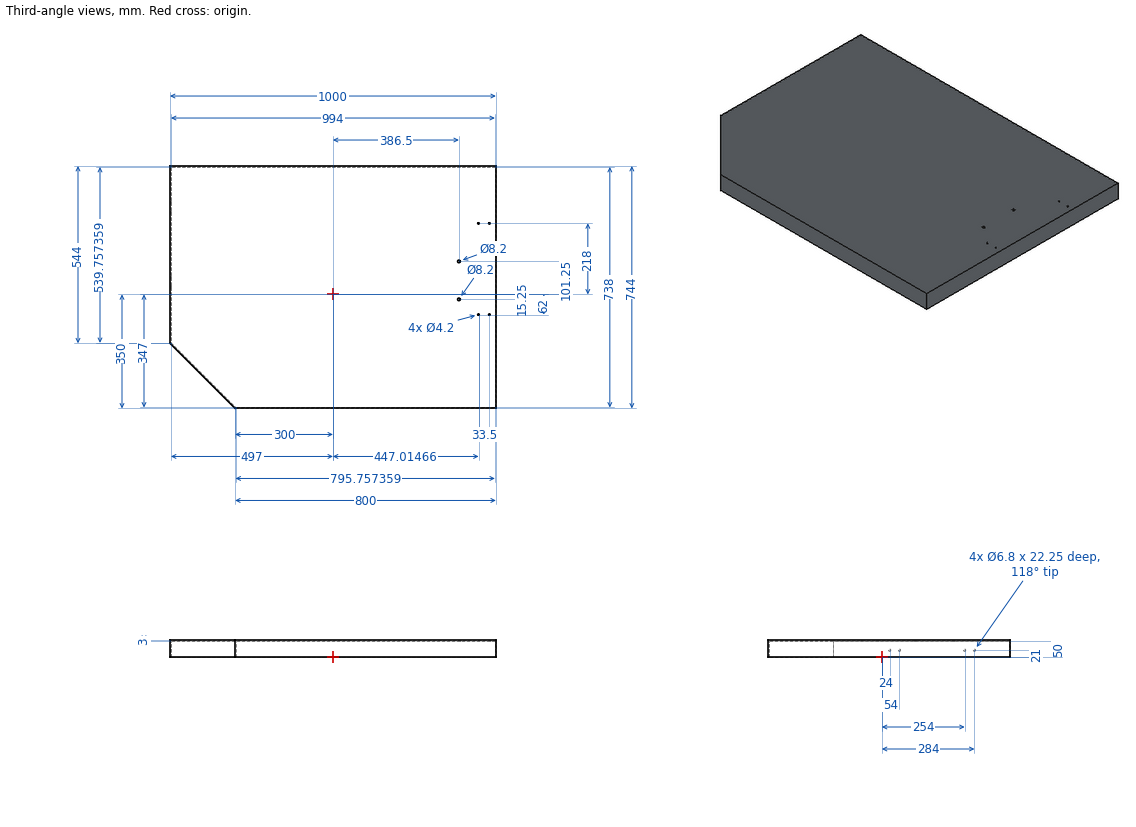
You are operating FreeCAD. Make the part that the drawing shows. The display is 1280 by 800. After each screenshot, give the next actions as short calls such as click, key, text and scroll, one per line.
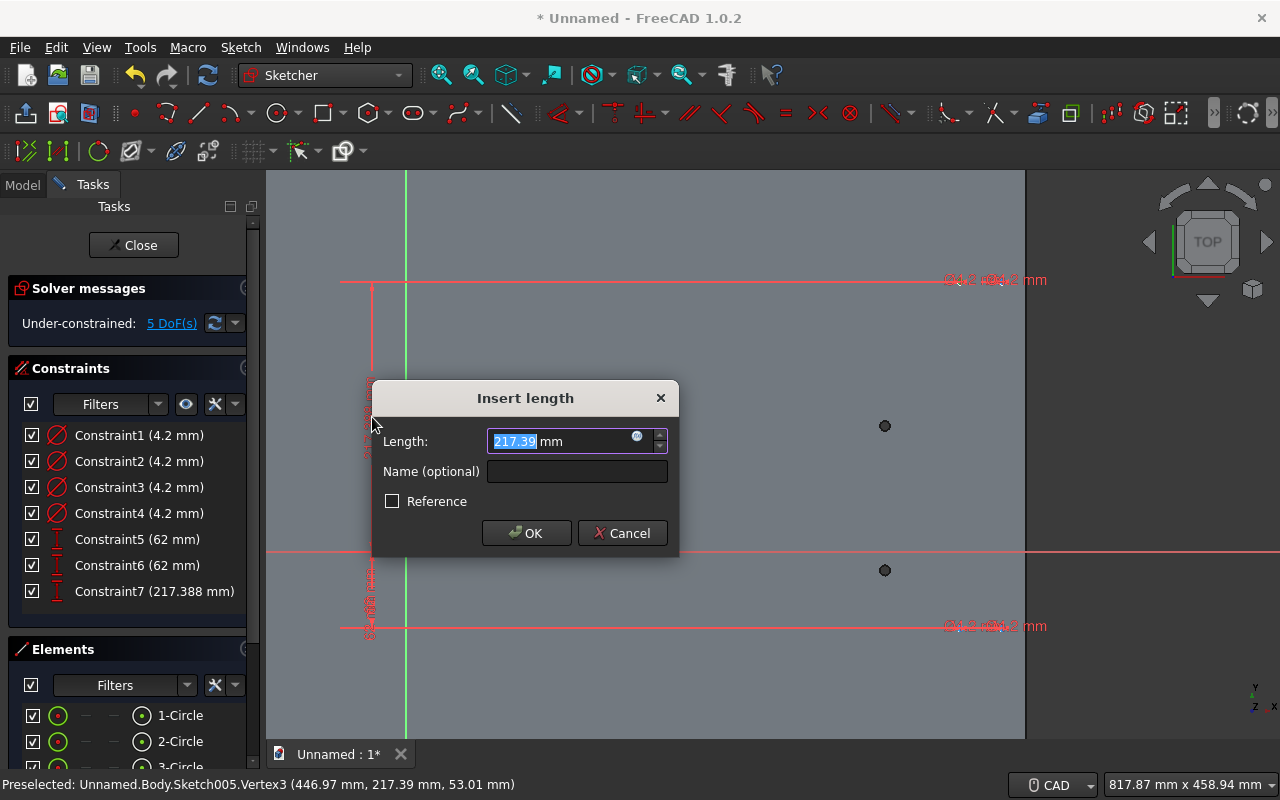
text(218)
key(Return)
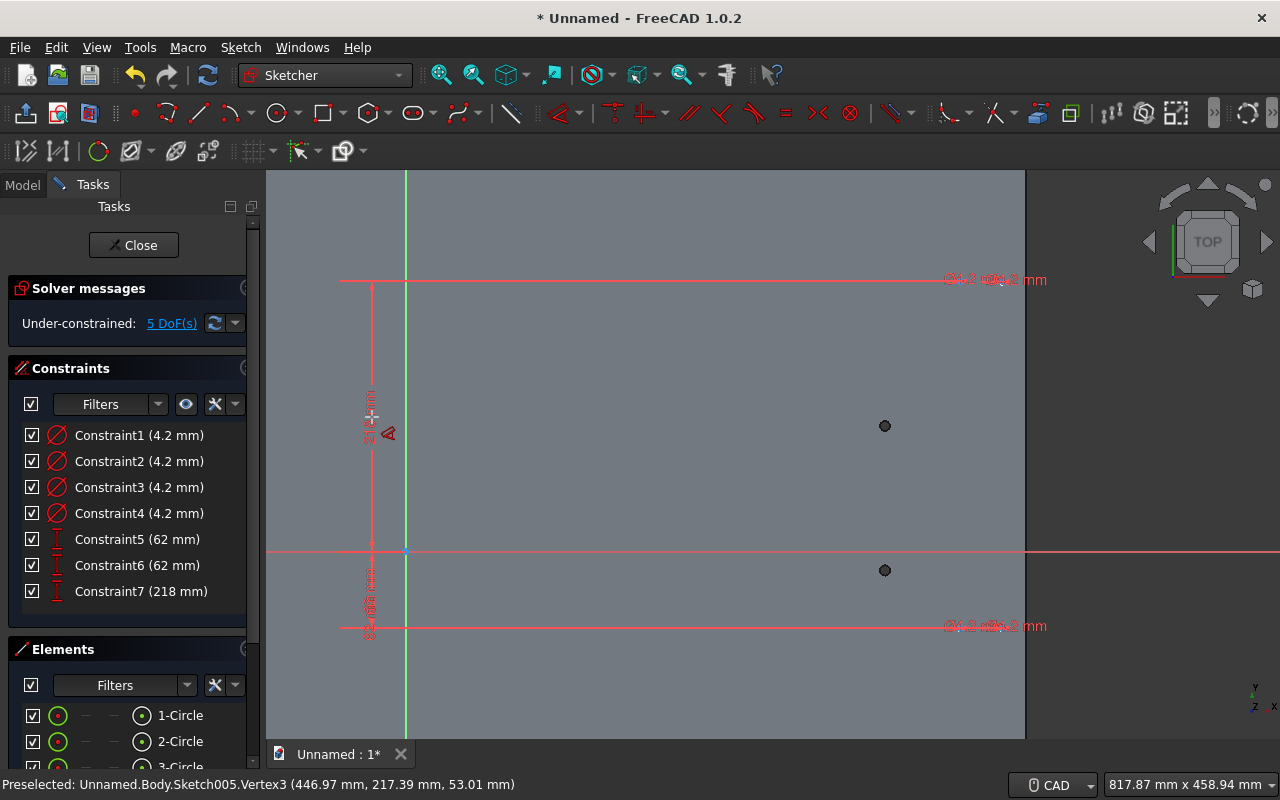
click(1002, 282)
click(372, 355)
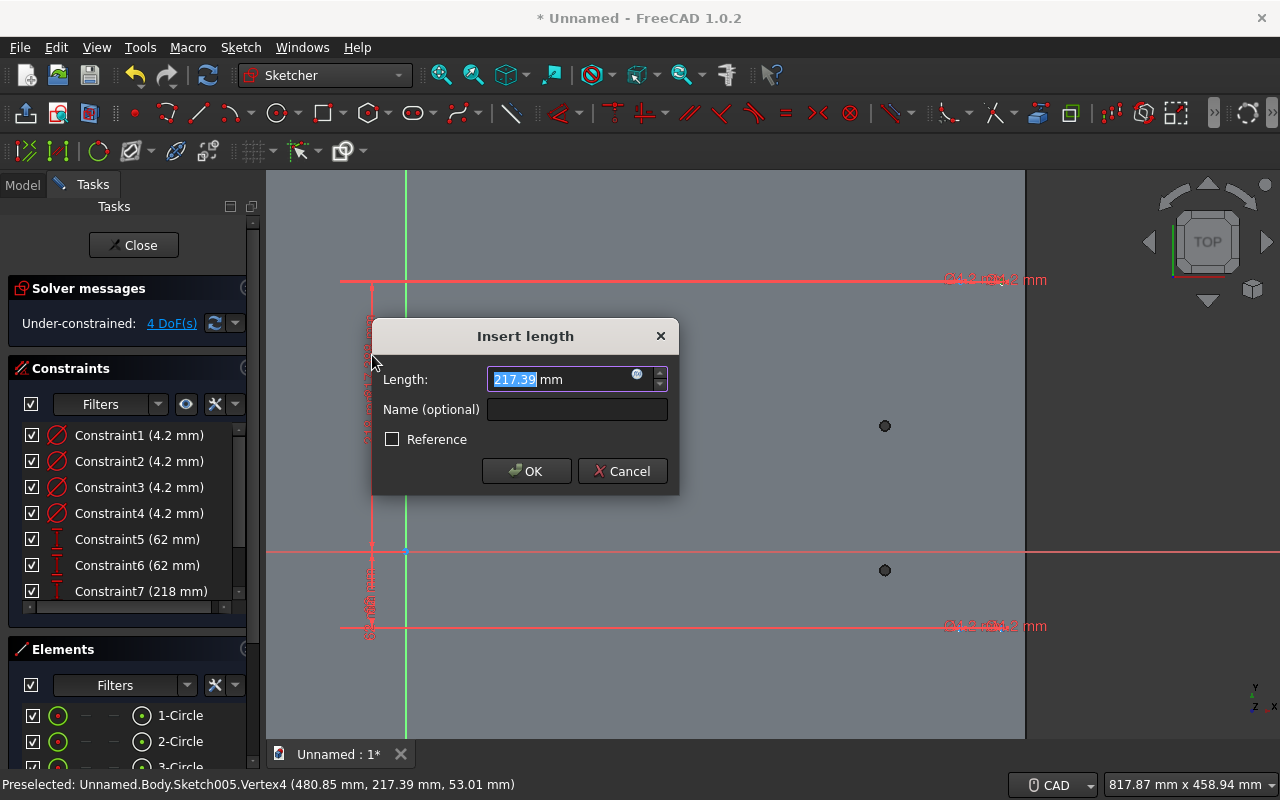
text(218)
key(Return)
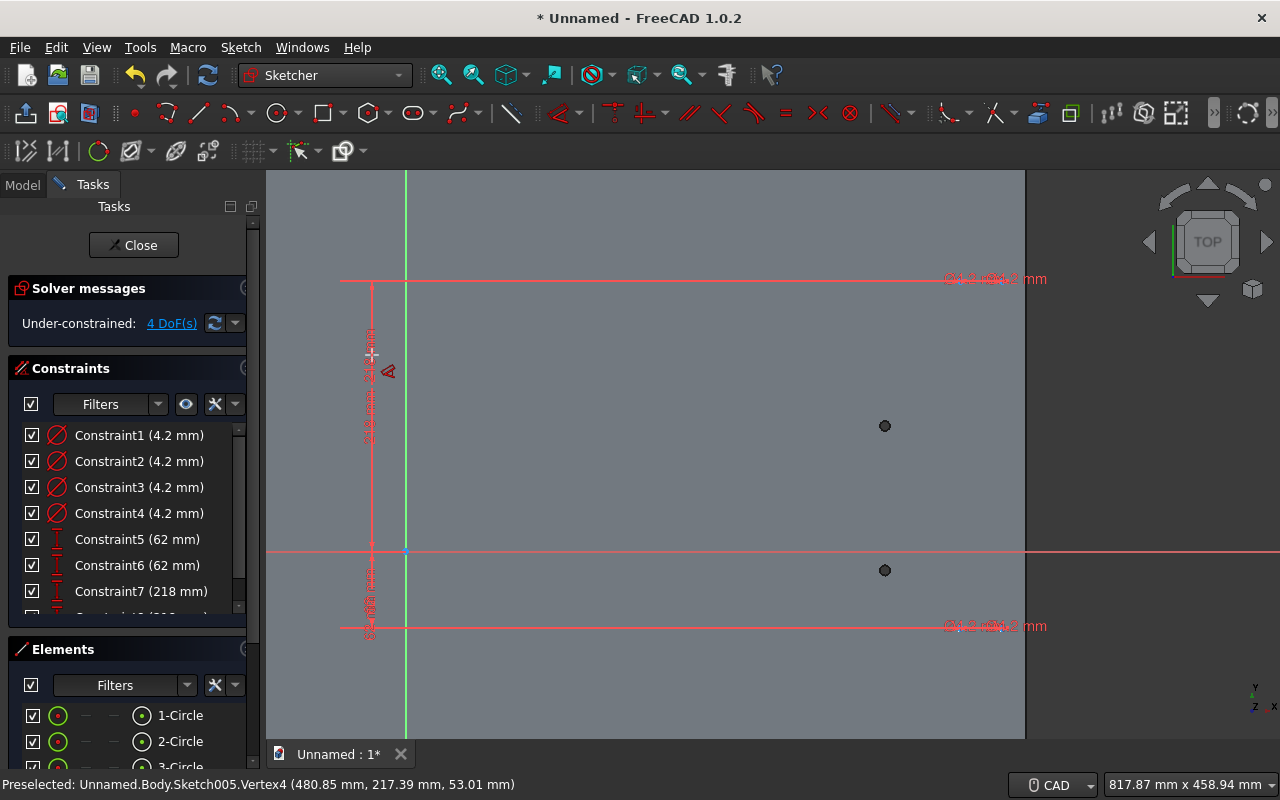
click(960, 628)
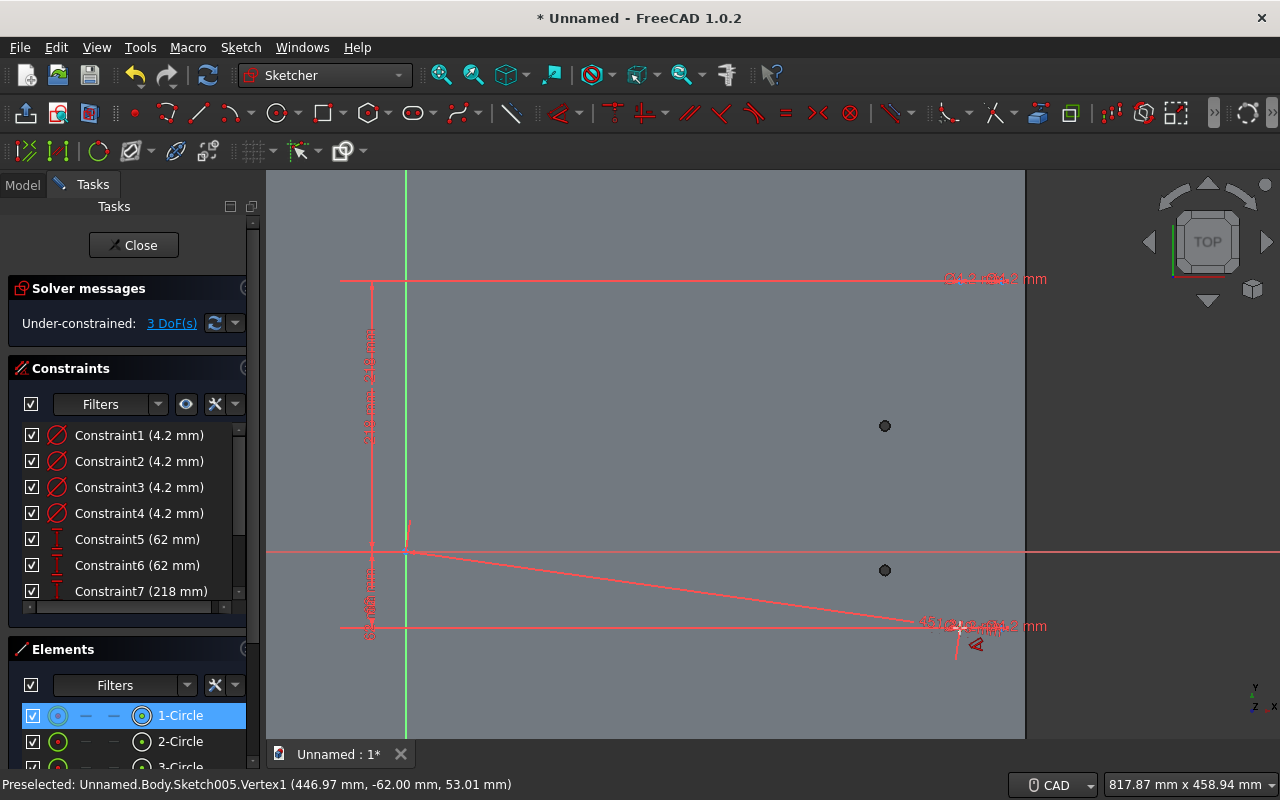
click(1002, 628)
click(981, 662)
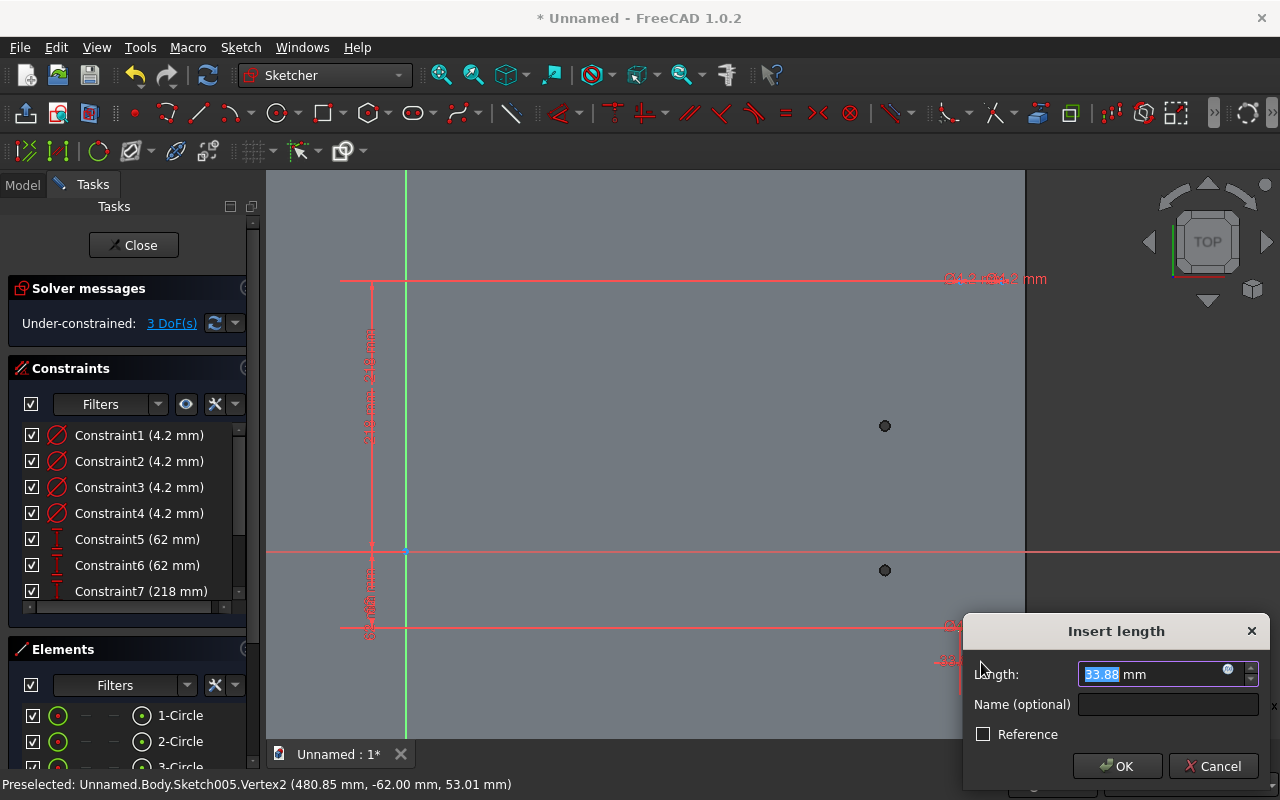
text(33.5)
key(Return)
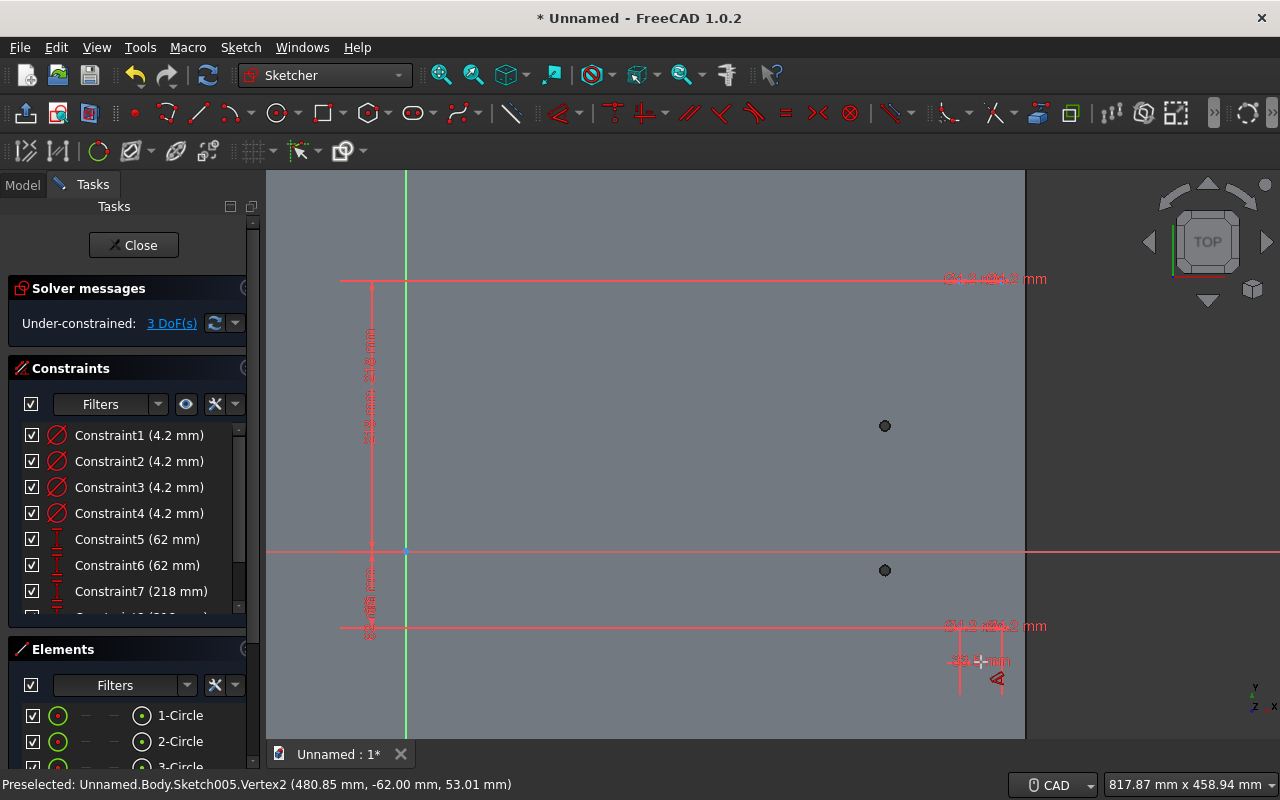
click(1002, 628)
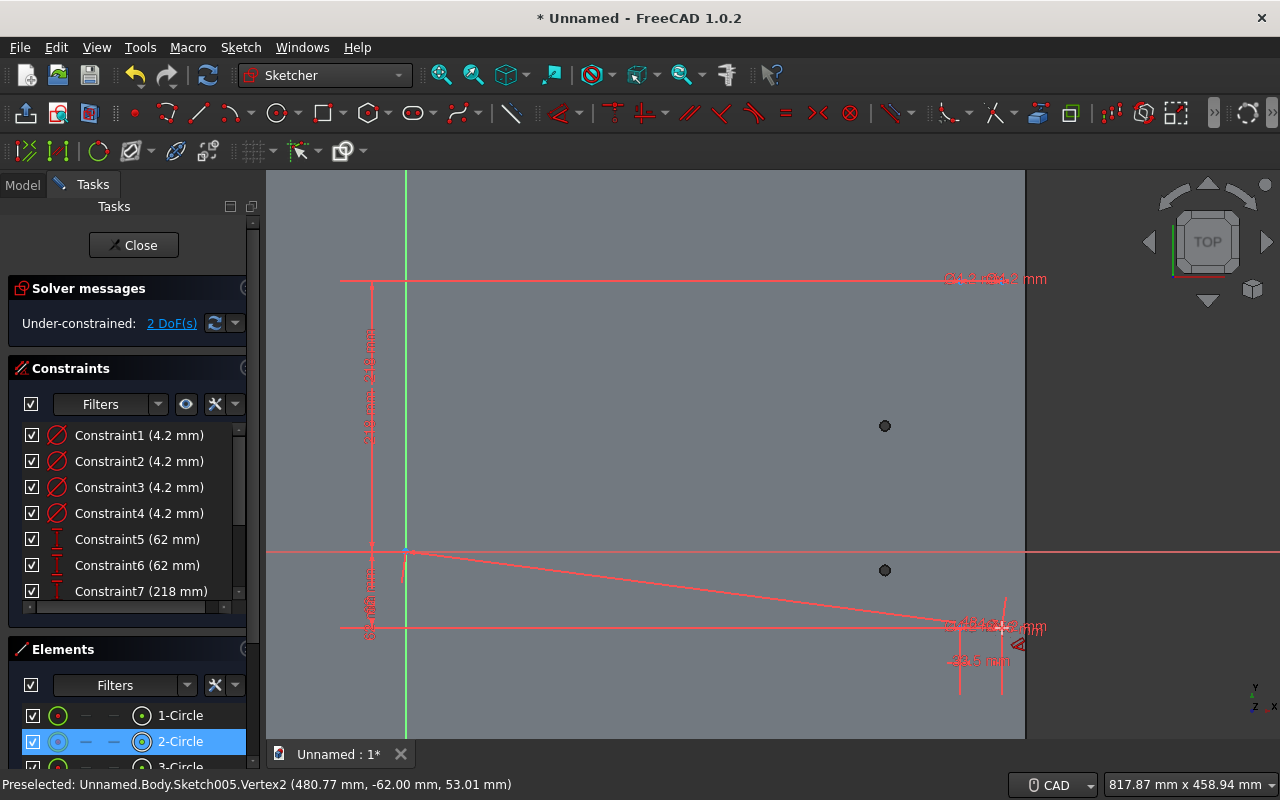
click(960, 281)
click(981, 247)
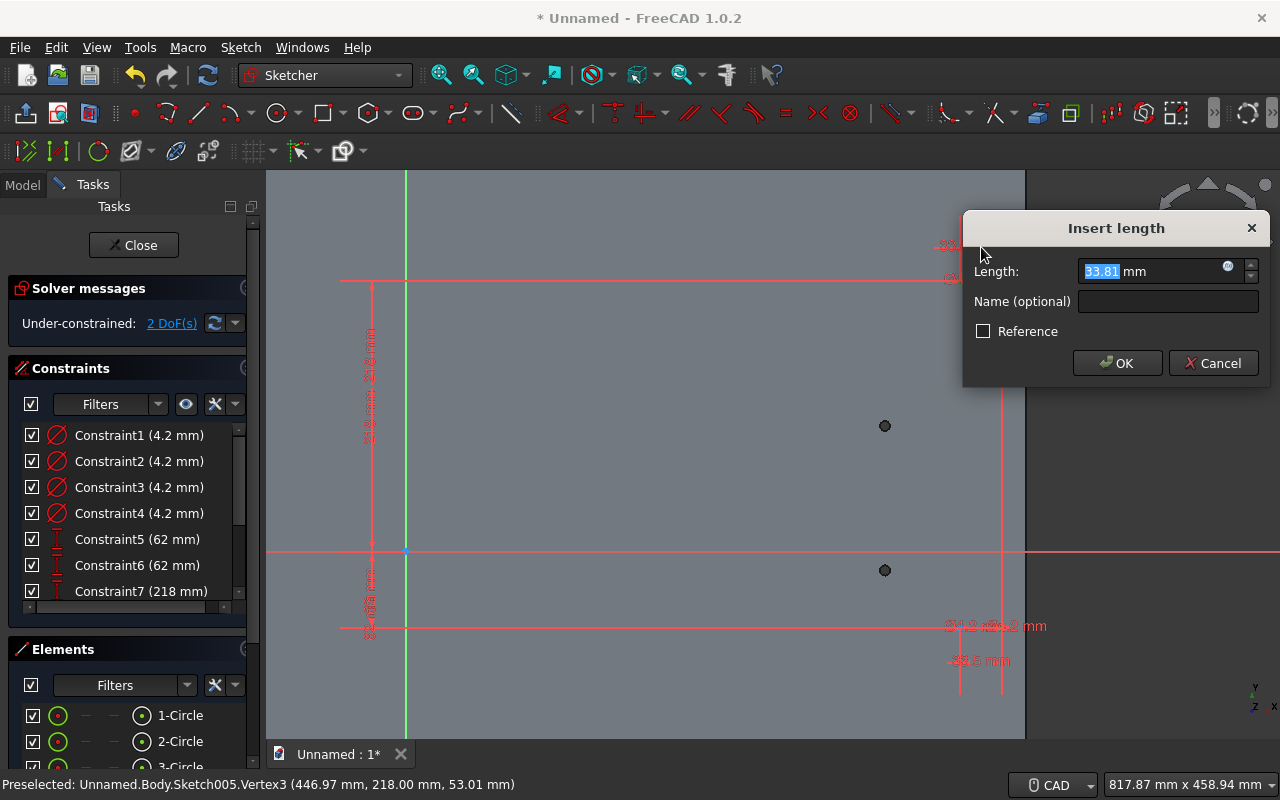
text(33.5)
key(Return)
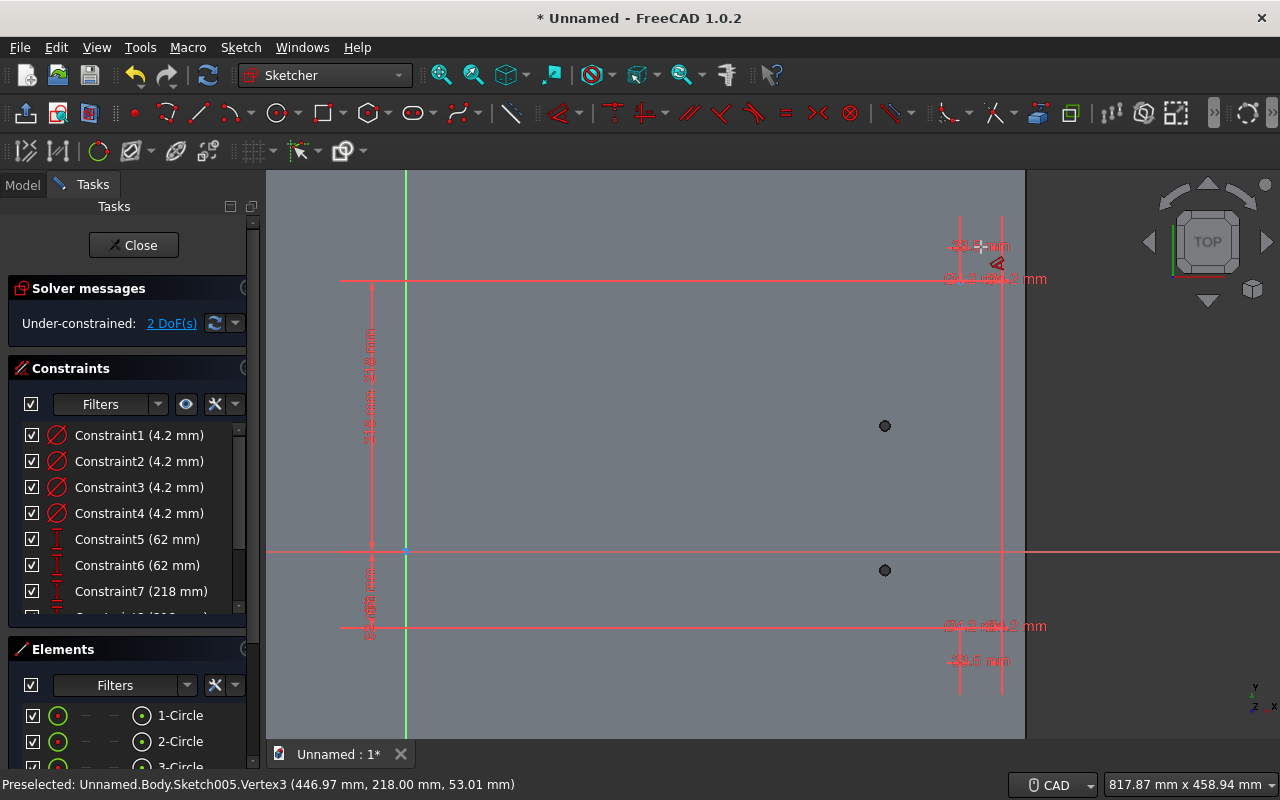
click(960, 281)